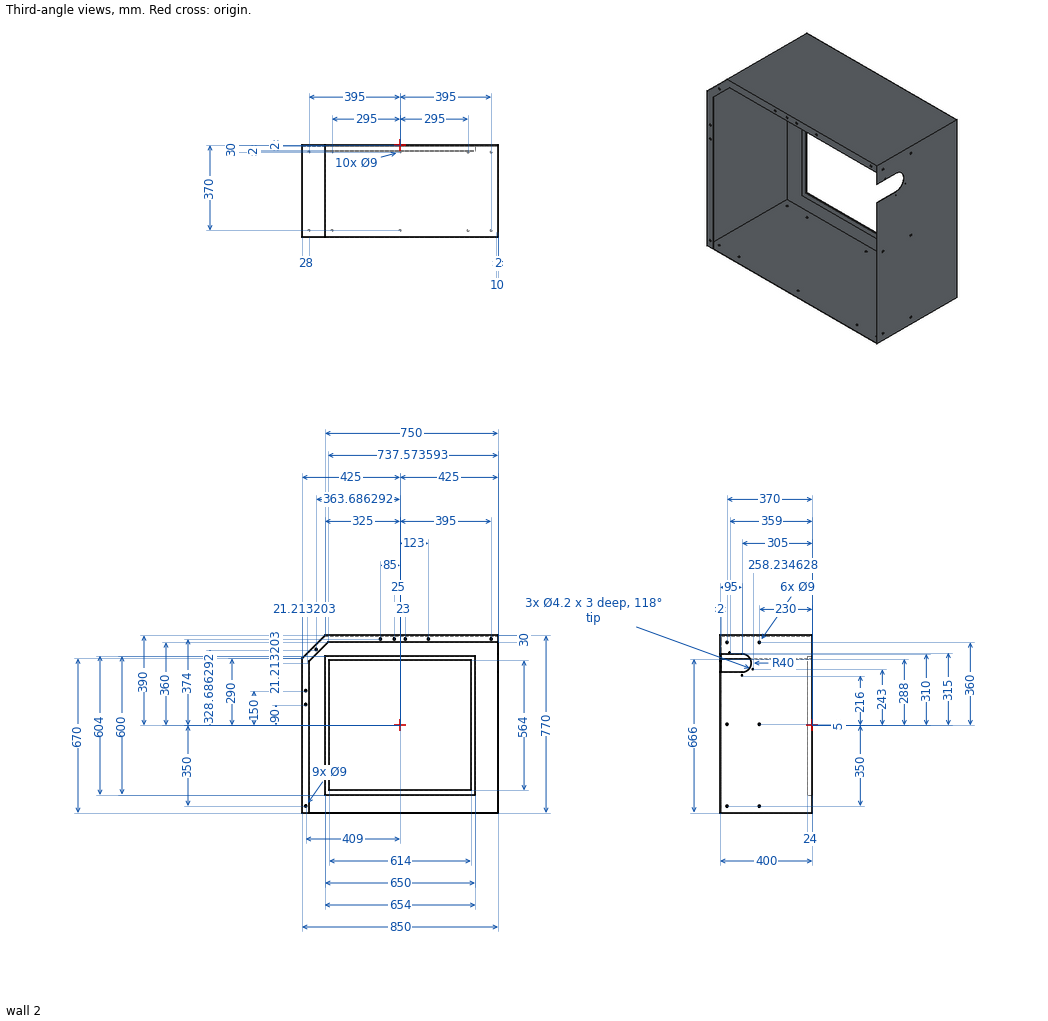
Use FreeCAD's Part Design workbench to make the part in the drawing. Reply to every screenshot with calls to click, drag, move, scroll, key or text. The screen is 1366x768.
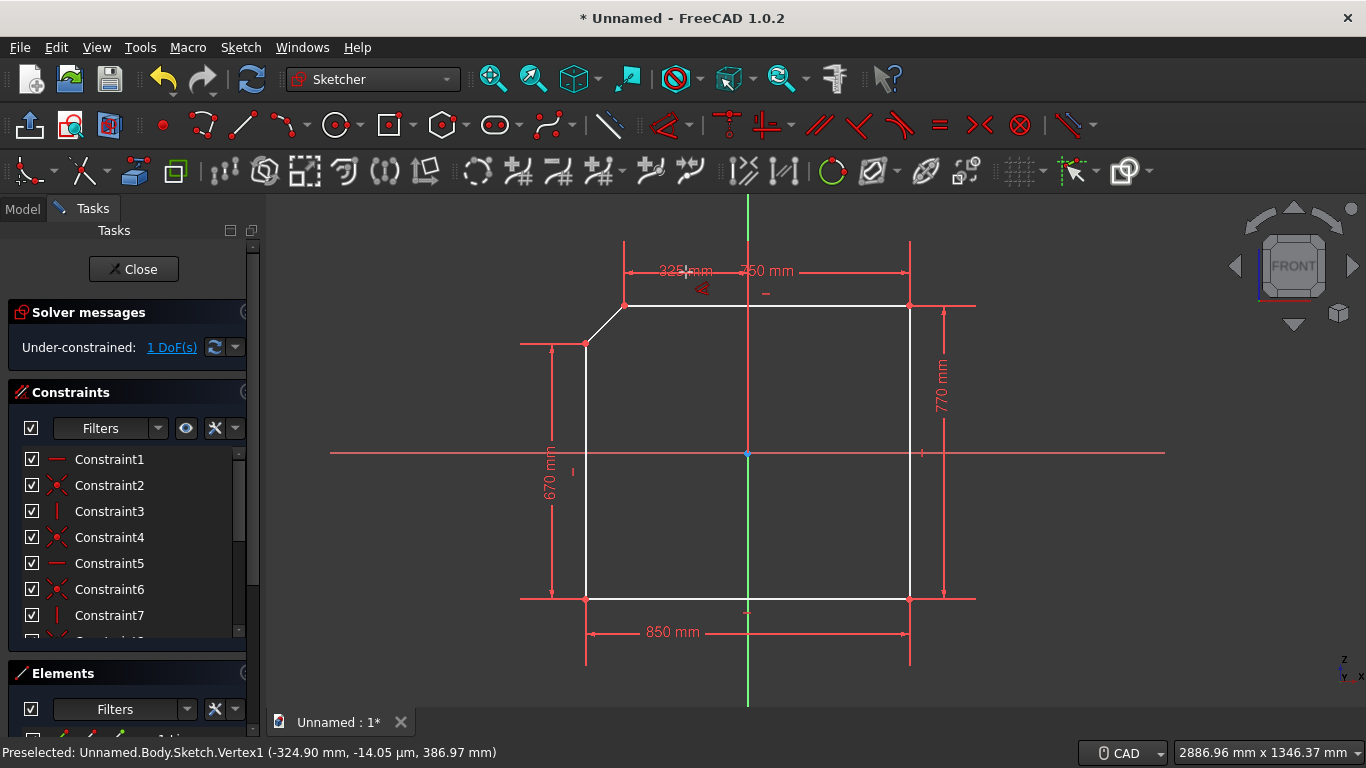
click(624, 306)
click(782, 380)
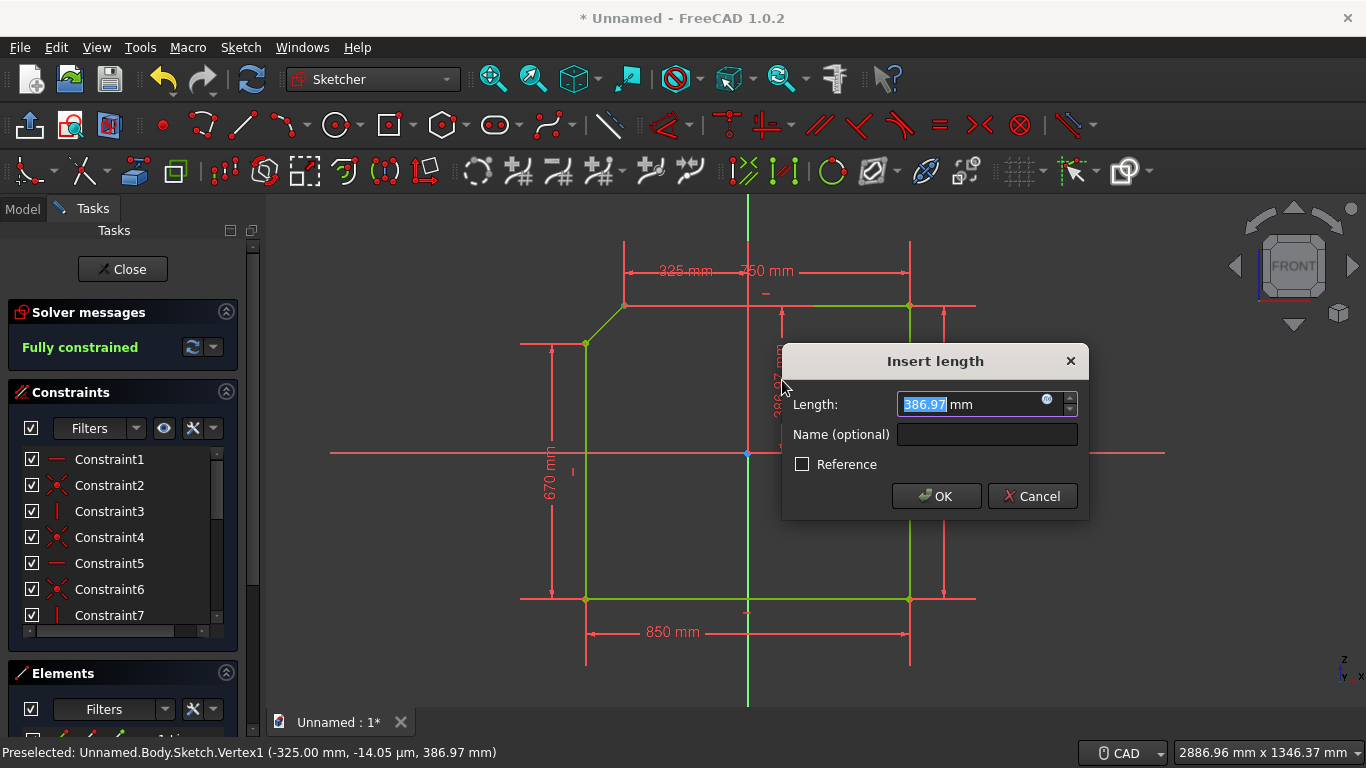
text(390)
key(Return)
key(Escape)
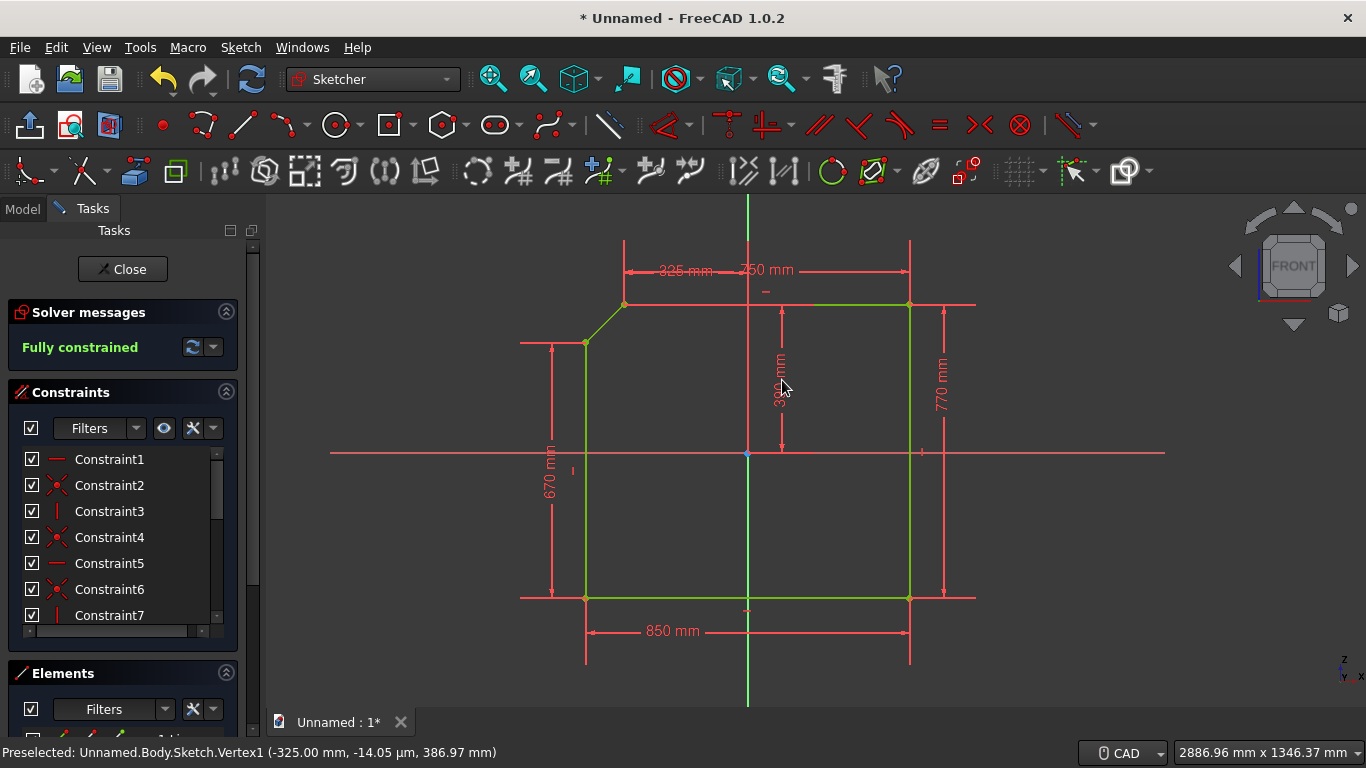
click(123, 269)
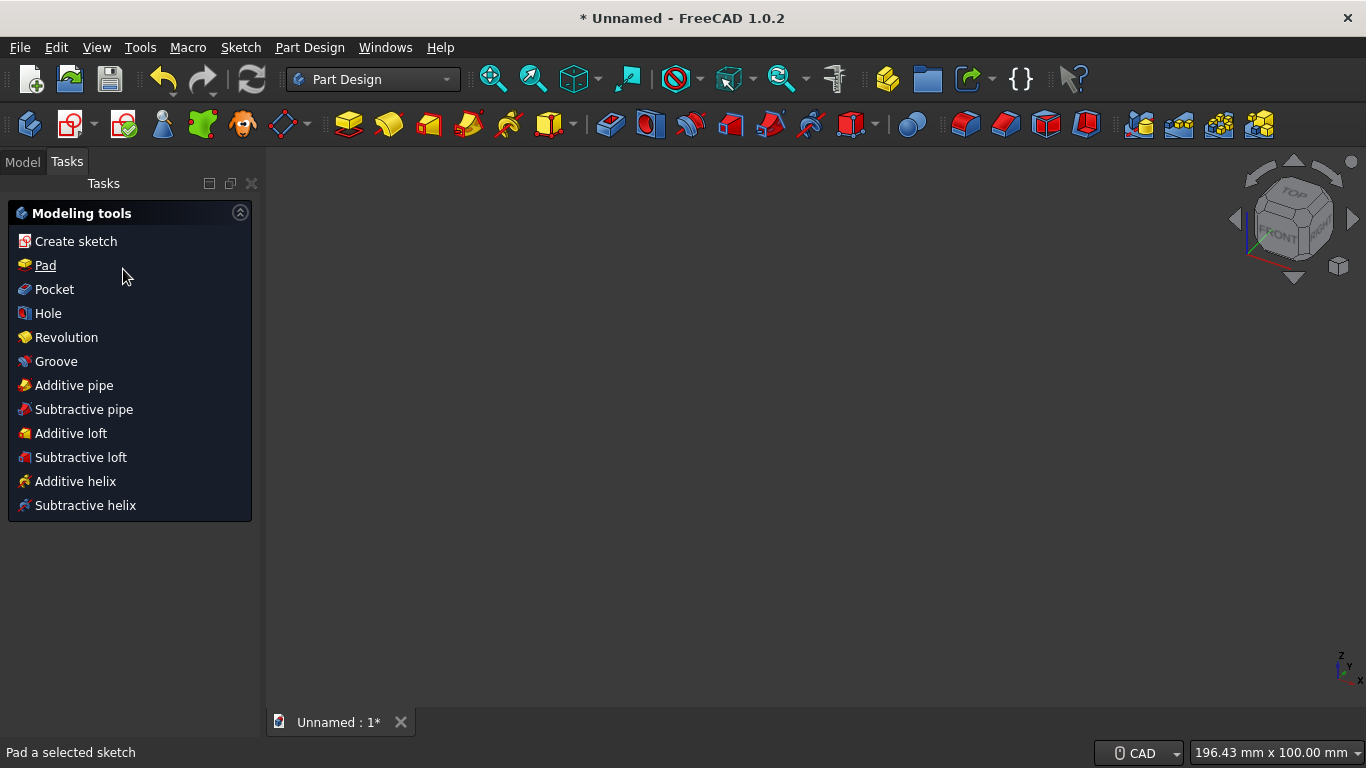
click(350, 124)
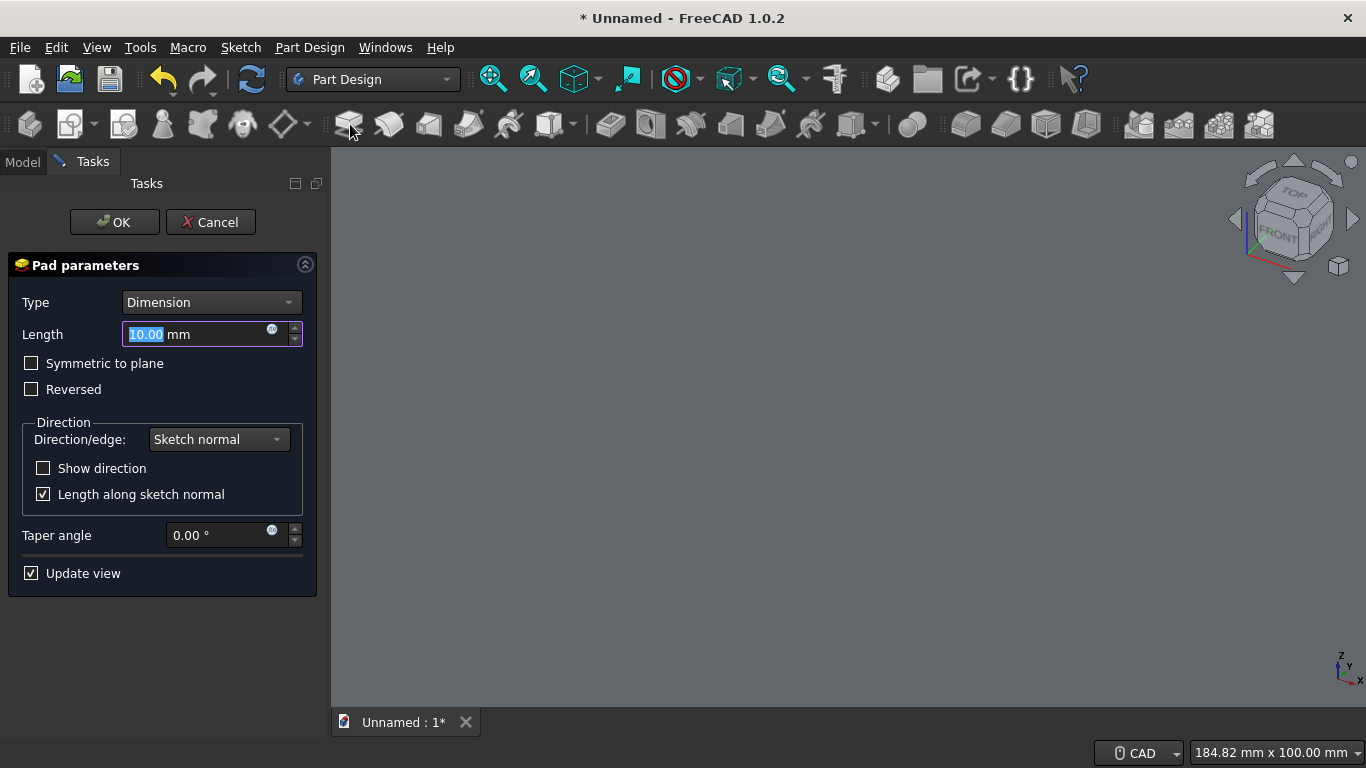
text(400)
key(Tab)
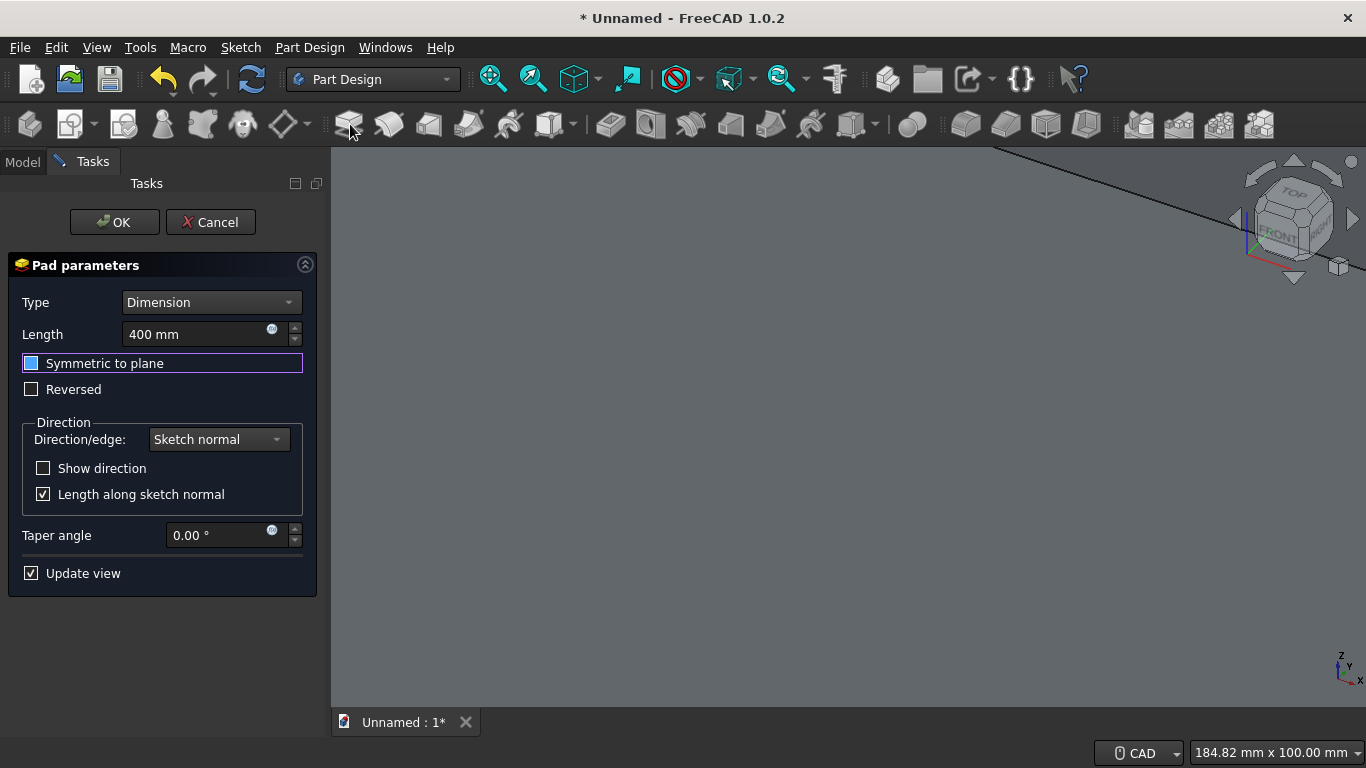
click(115, 222)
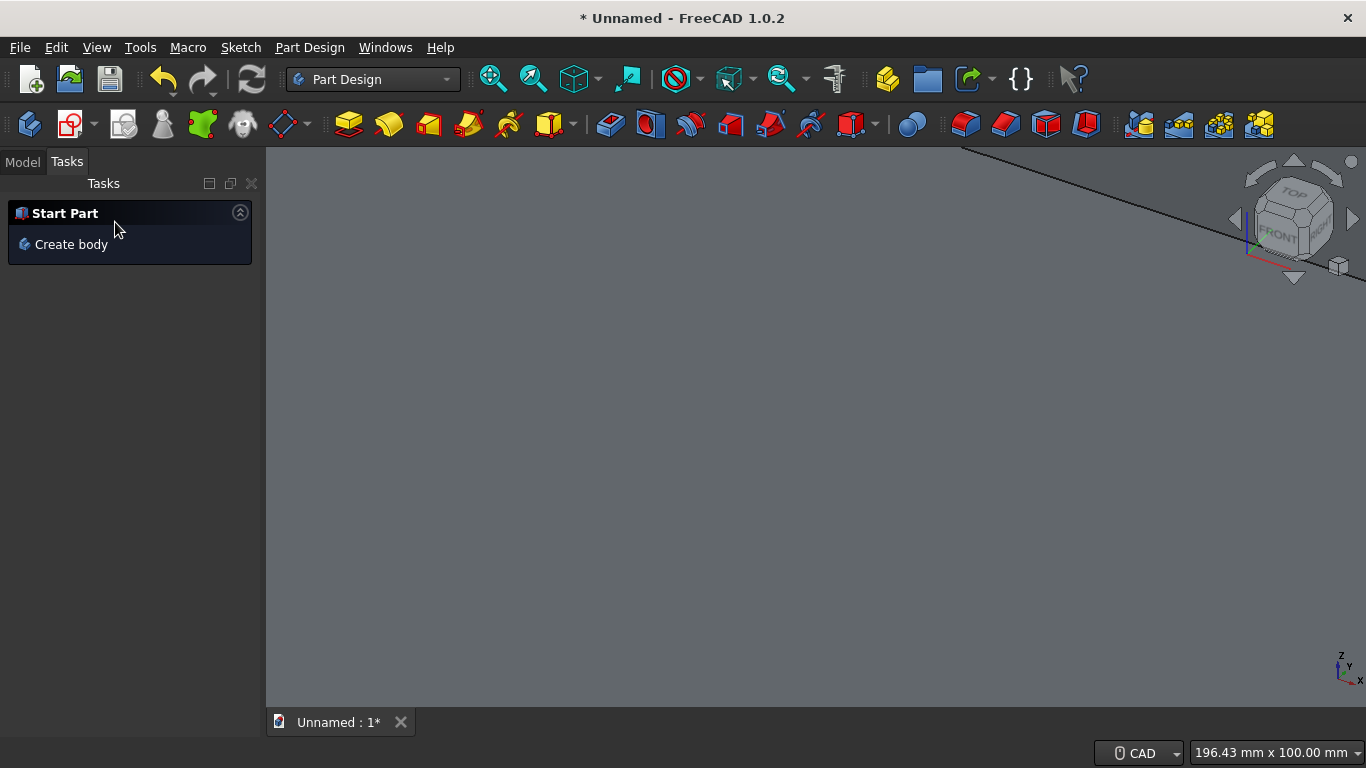
click(494, 80)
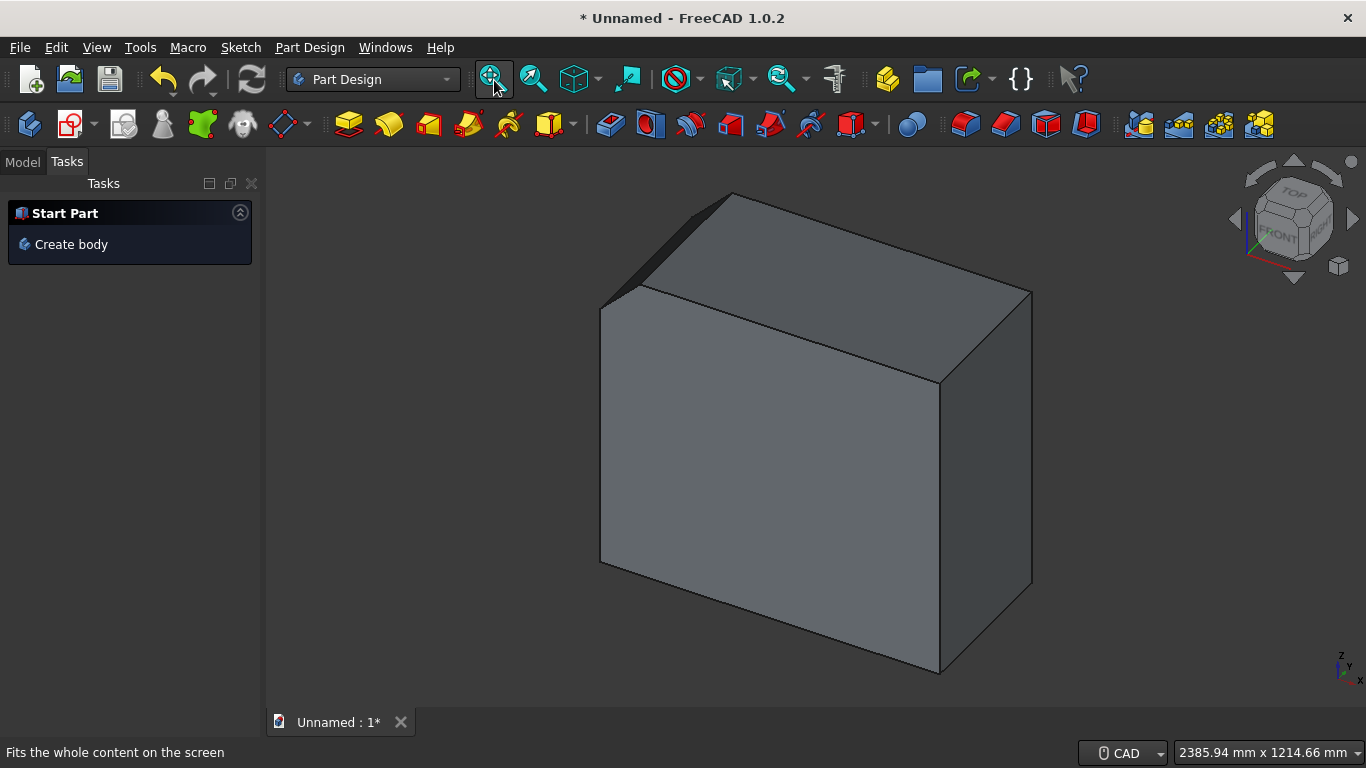
click(770, 472)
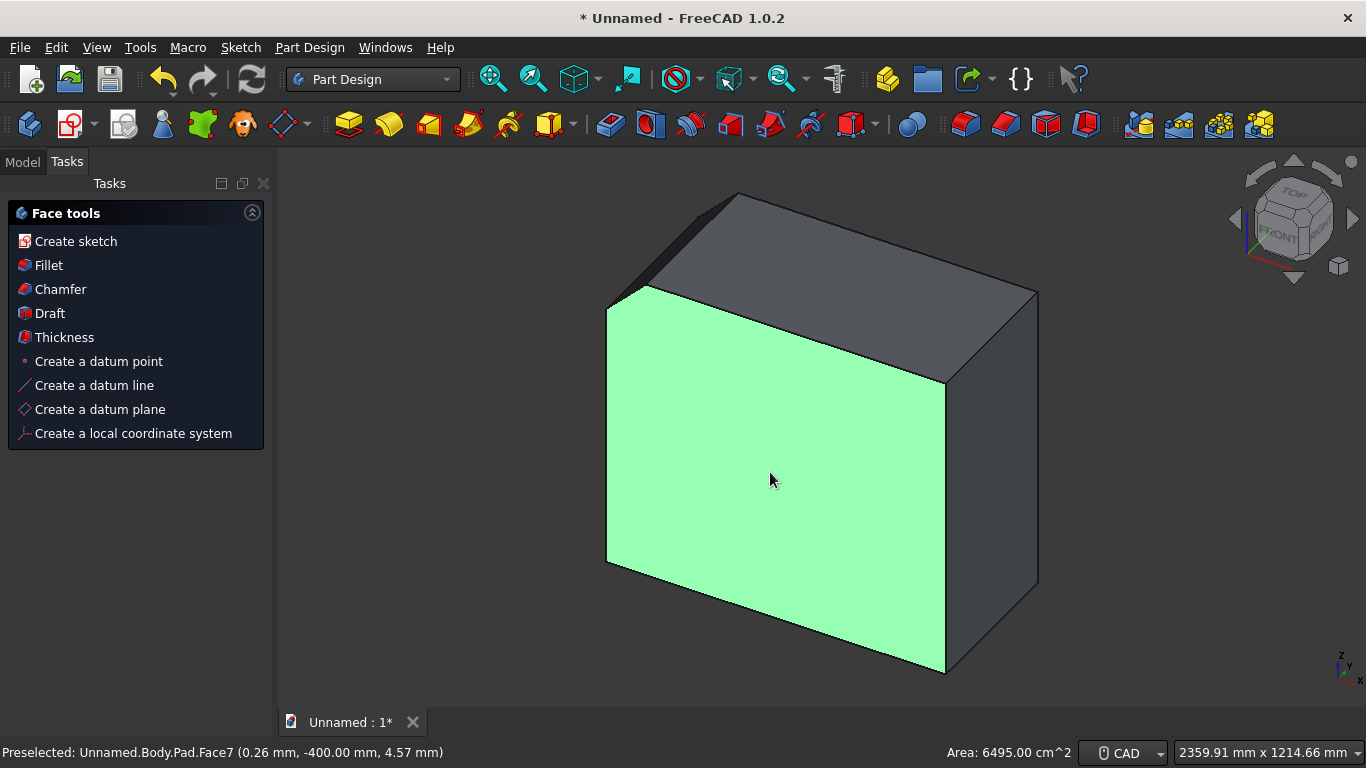
click(1086, 124)